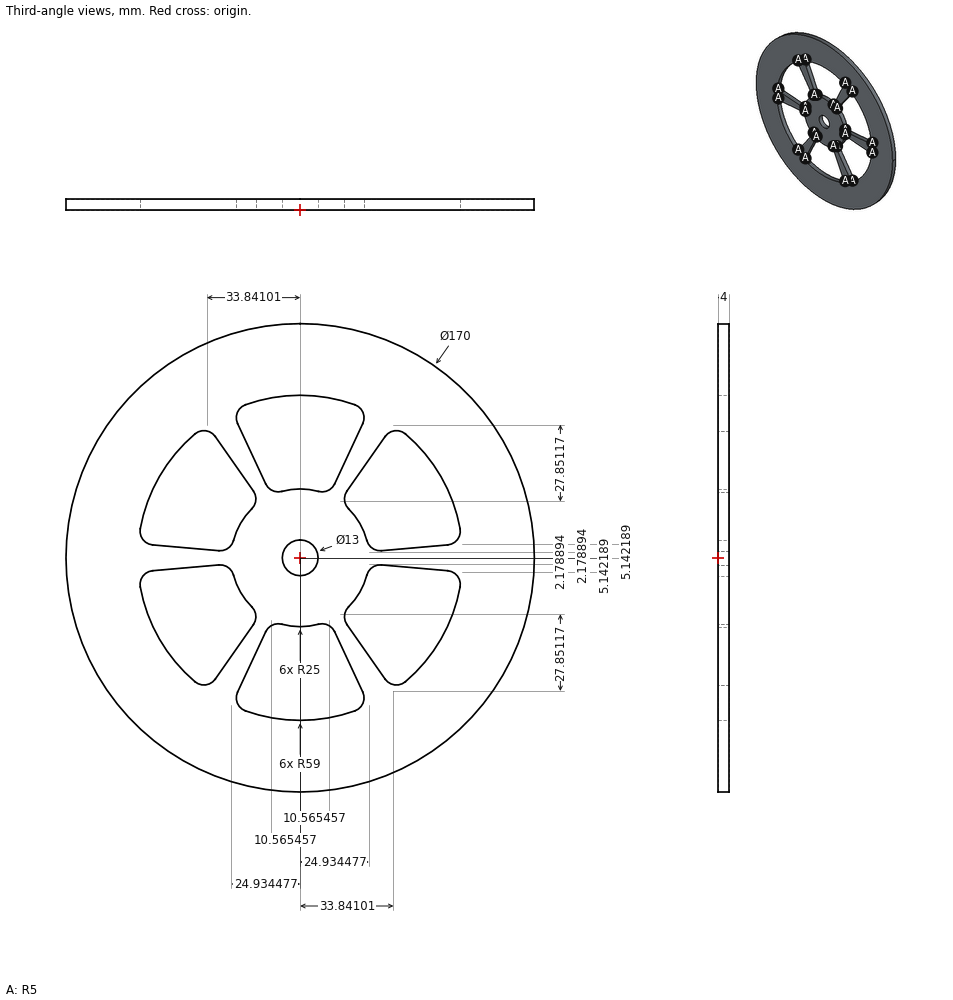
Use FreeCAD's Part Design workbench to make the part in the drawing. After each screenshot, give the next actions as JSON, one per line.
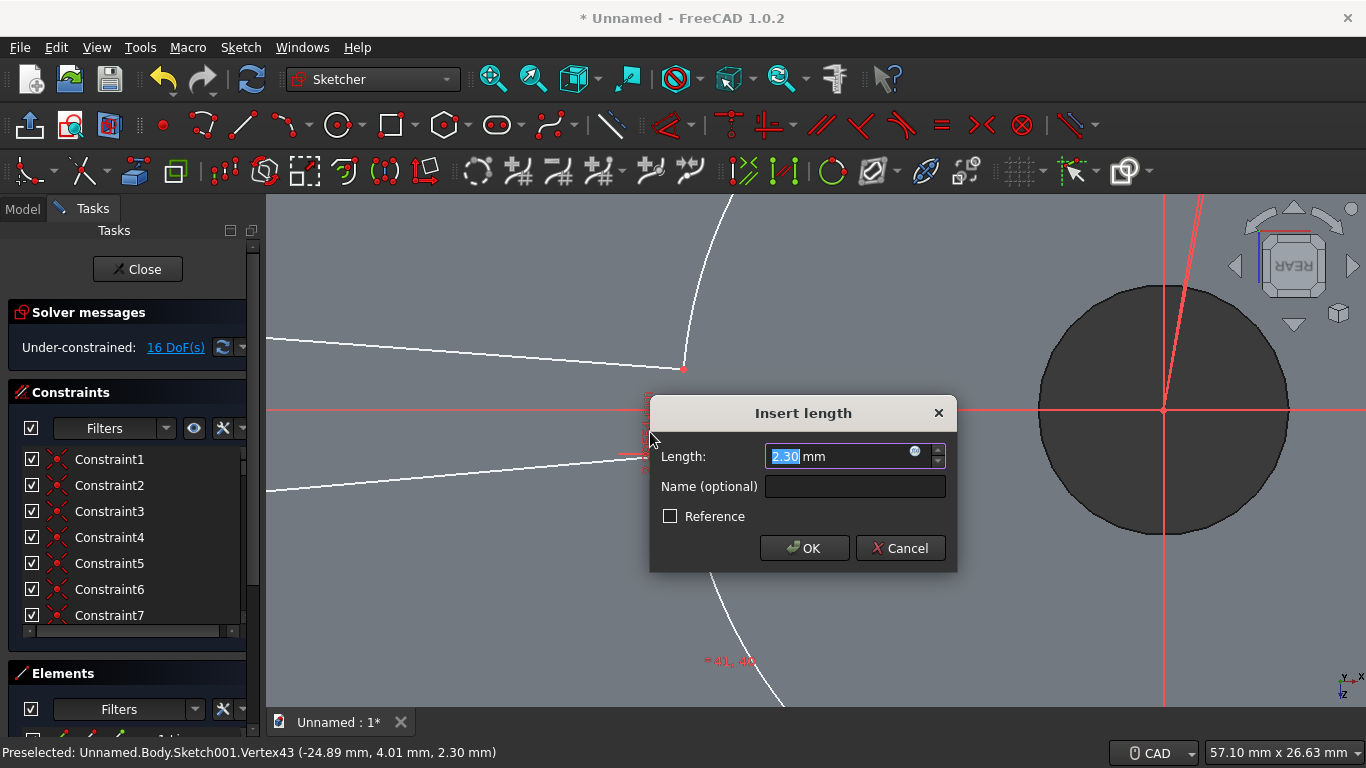
{"action": "type", "text": "2.178894"}
{"action": "key", "text": "Return"}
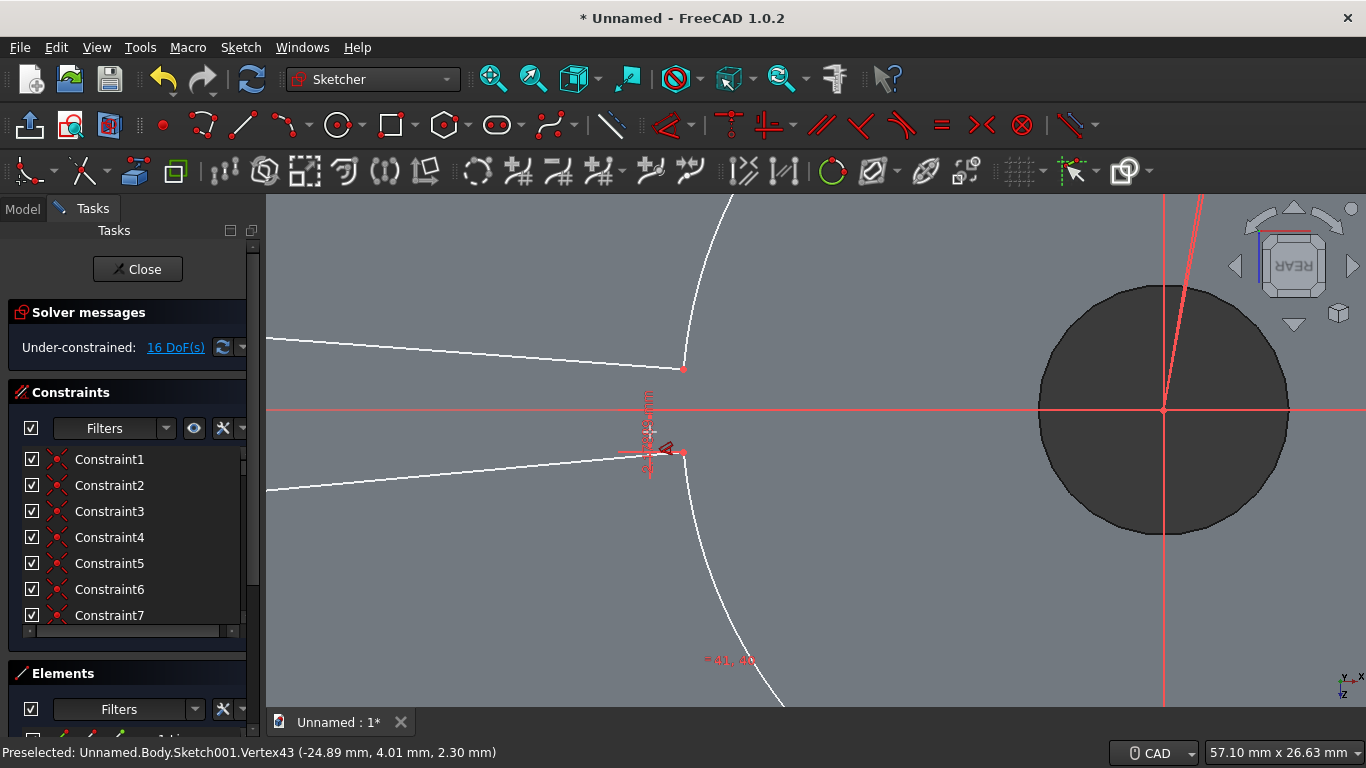
{"action": "scroll", "coordinate": [682, 457], "scroll_direction": "down", "scroll_amount": 10}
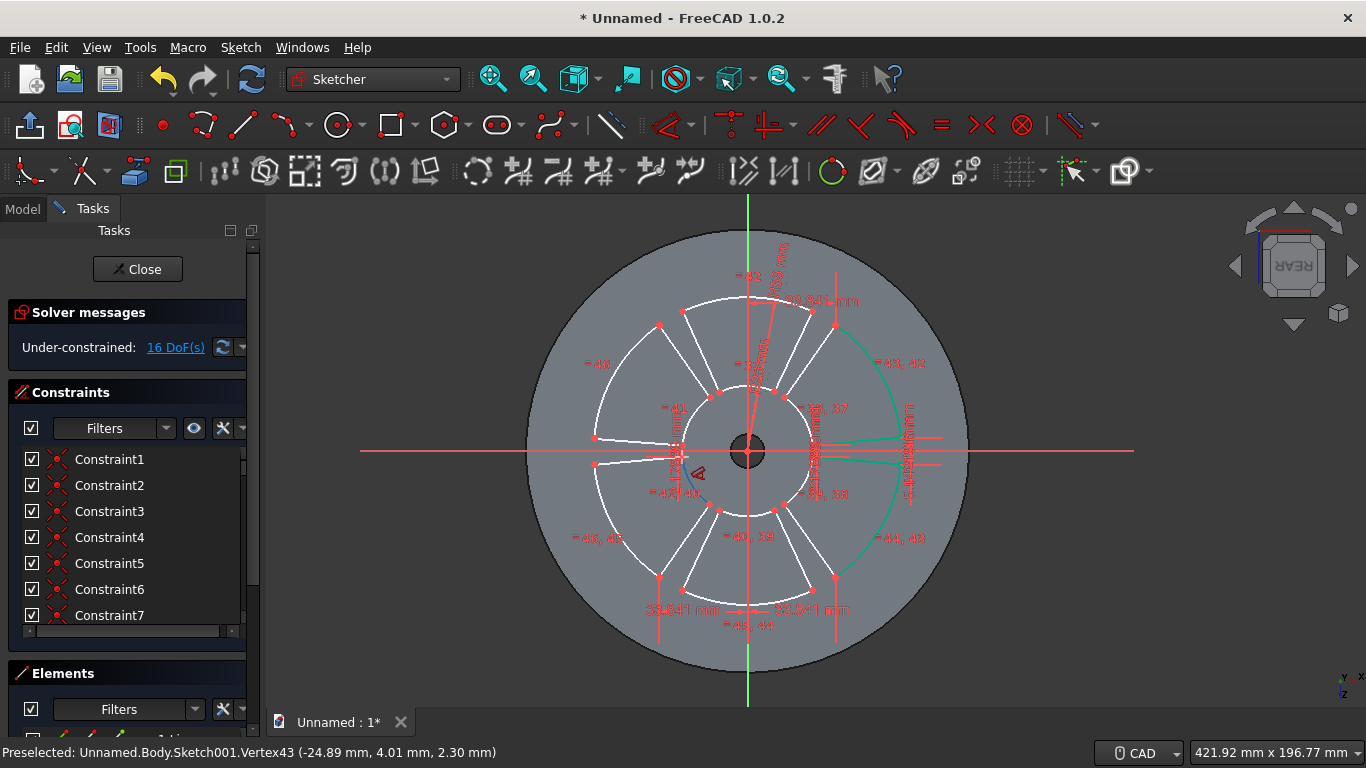
{"action": "scroll", "coordinate": [594, 465], "scroll_direction": "up", "scroll_amount": 6}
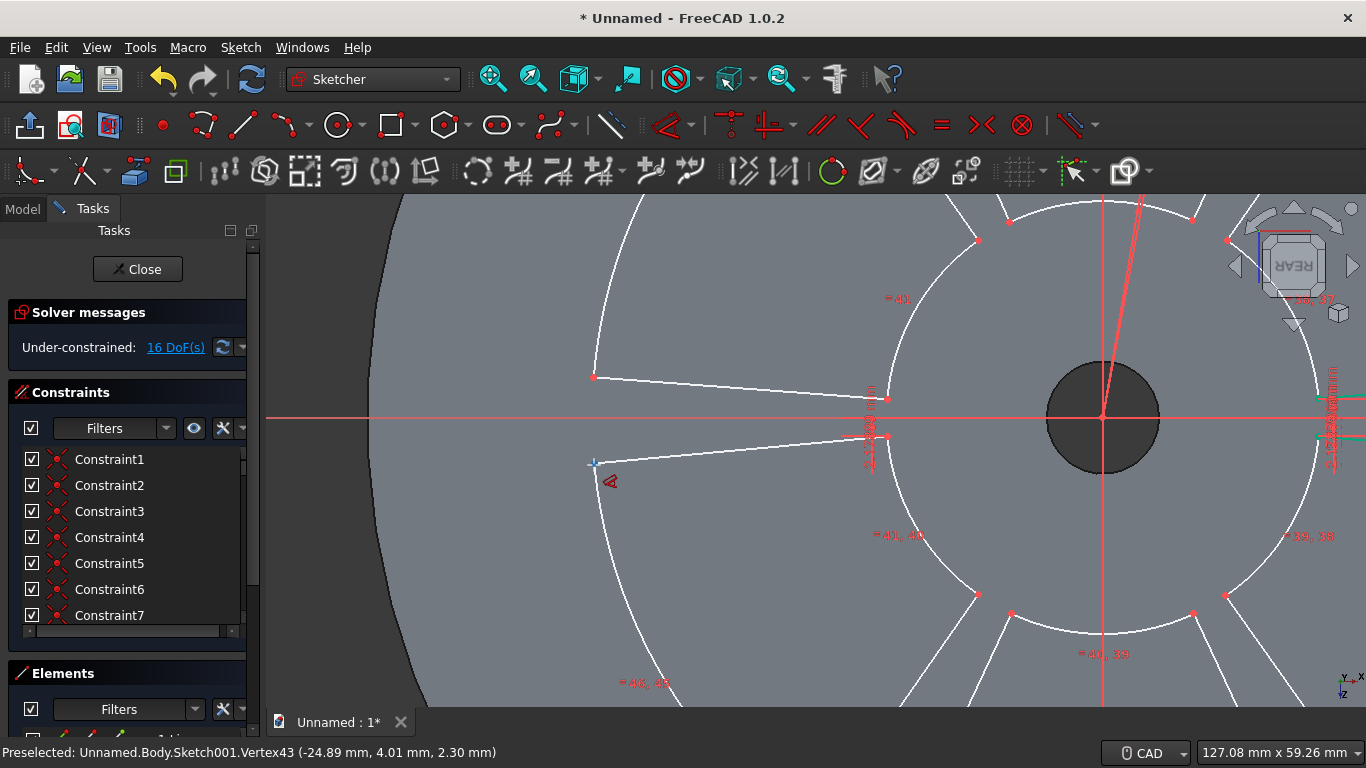
{"action": "left_click", "coordinate": [594, 463]}
{"action": "left_click", "coordinate": [560, 441]}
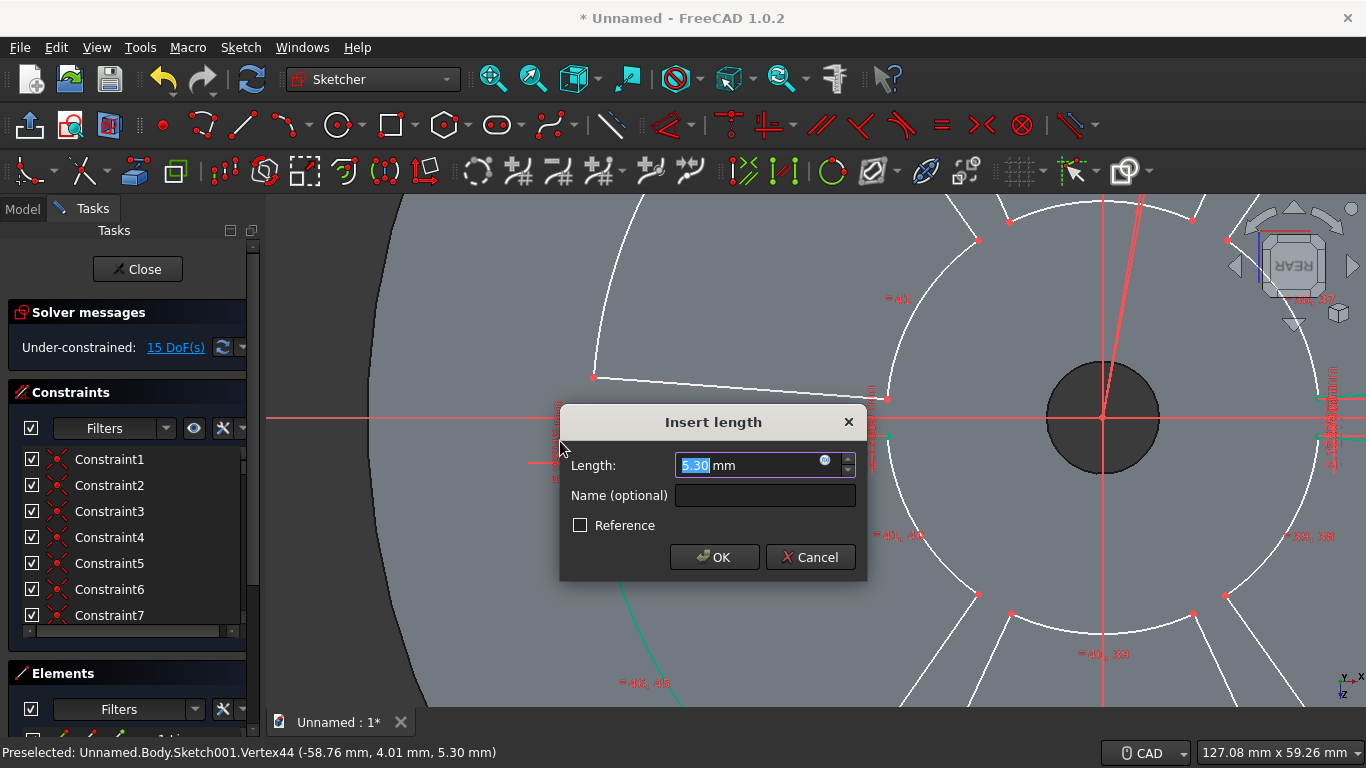
{"action": "type", "text": "5.142189"}
{"action": "key", "text": "Return"}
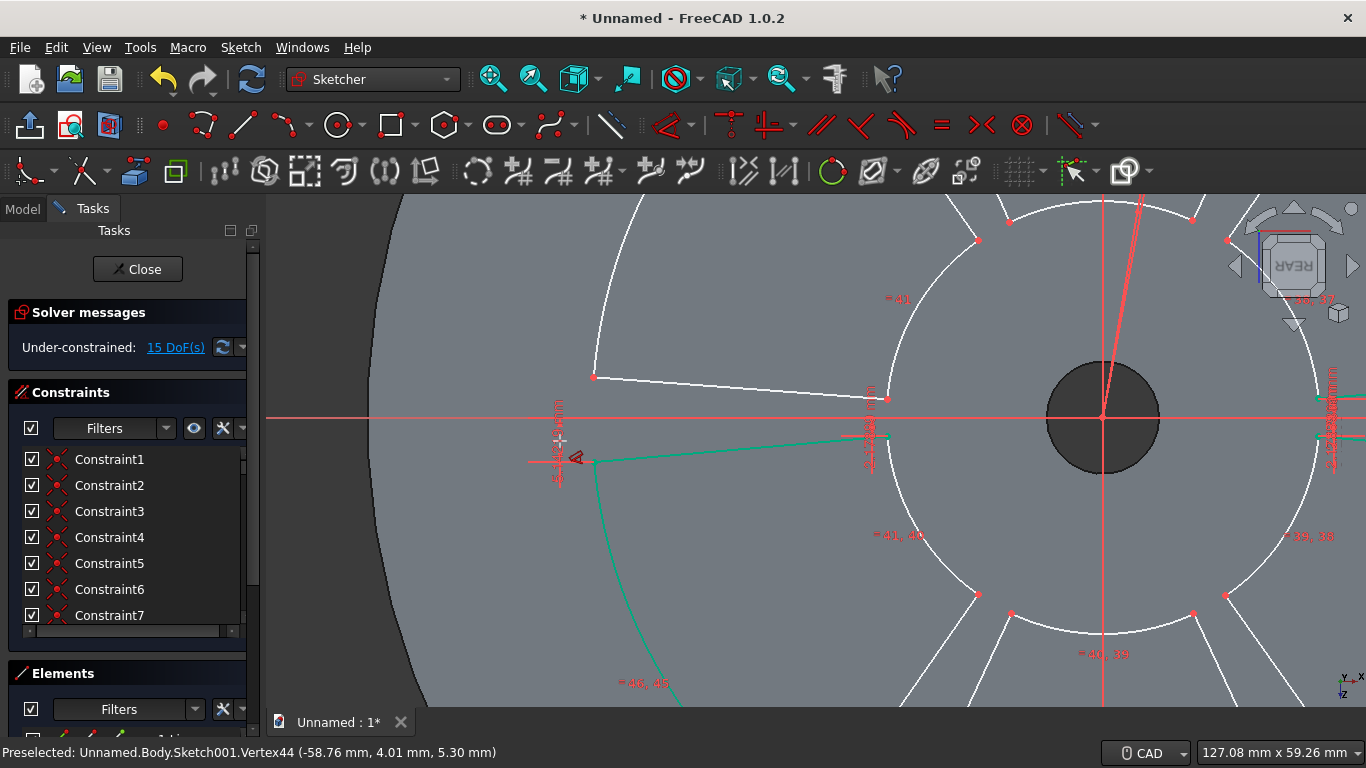
{"action": "left_click", "coordinate": [594, 377]}
{"action": "left_click", "coordinate": [560, 397]}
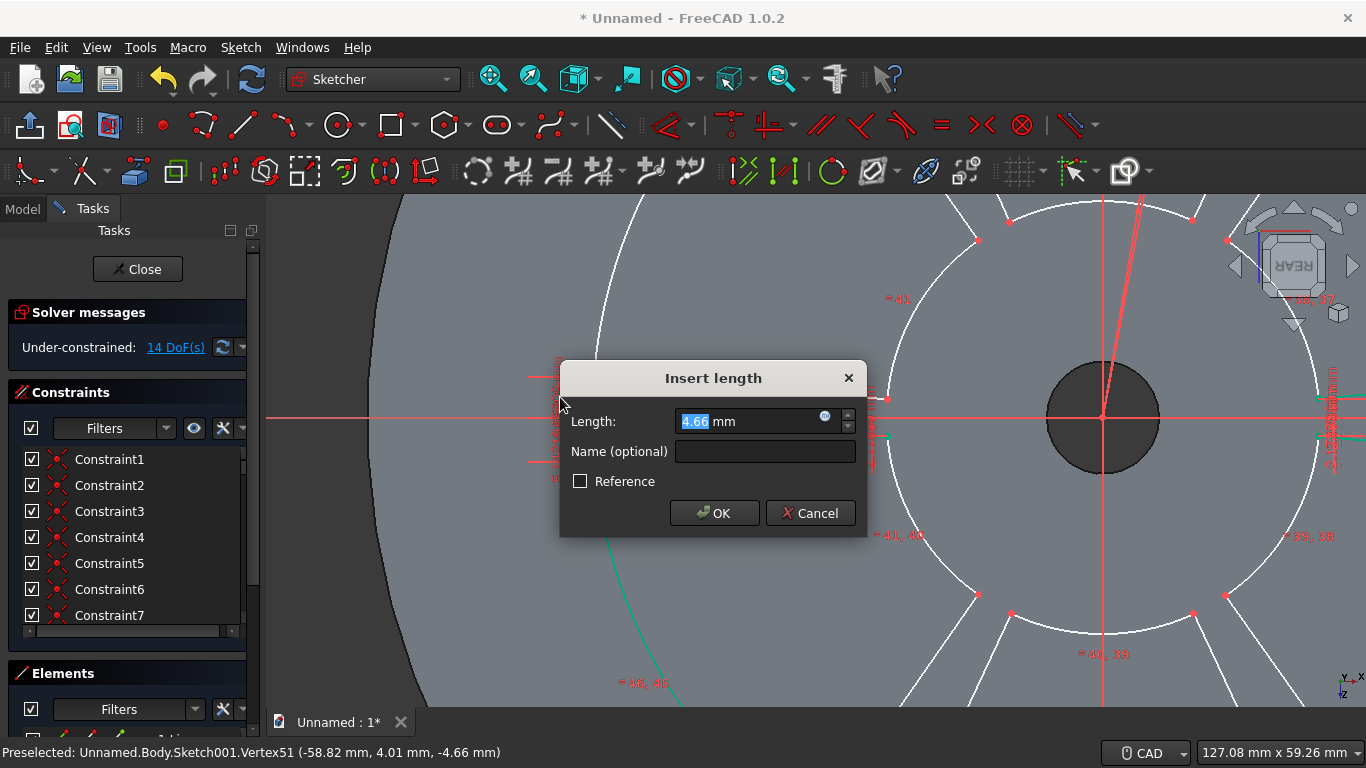
{"action": "type", "text": "5.142189"}
{"action": "key", "text": "Return"}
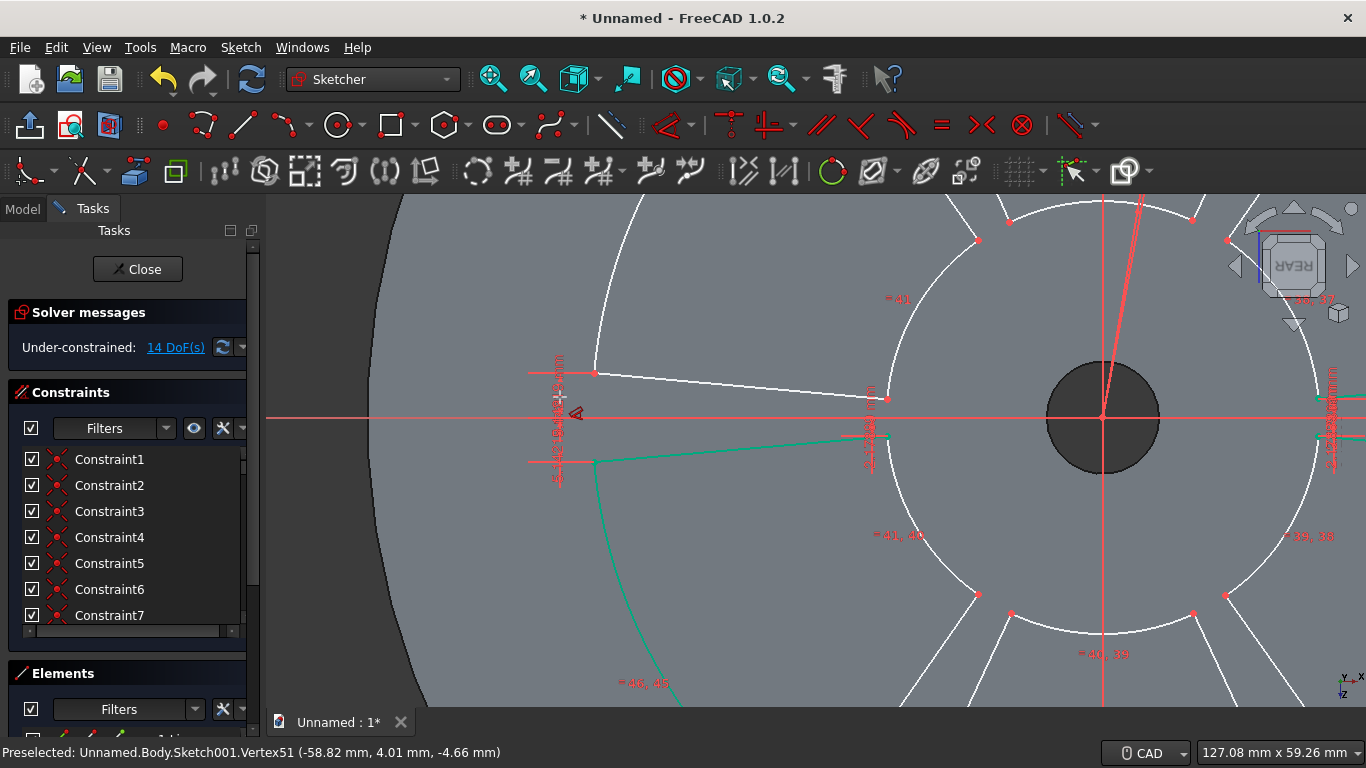
{"action": "scroll", "coordinate": [887, 399], "scroll_direction": "up", "scroll_amount": 4}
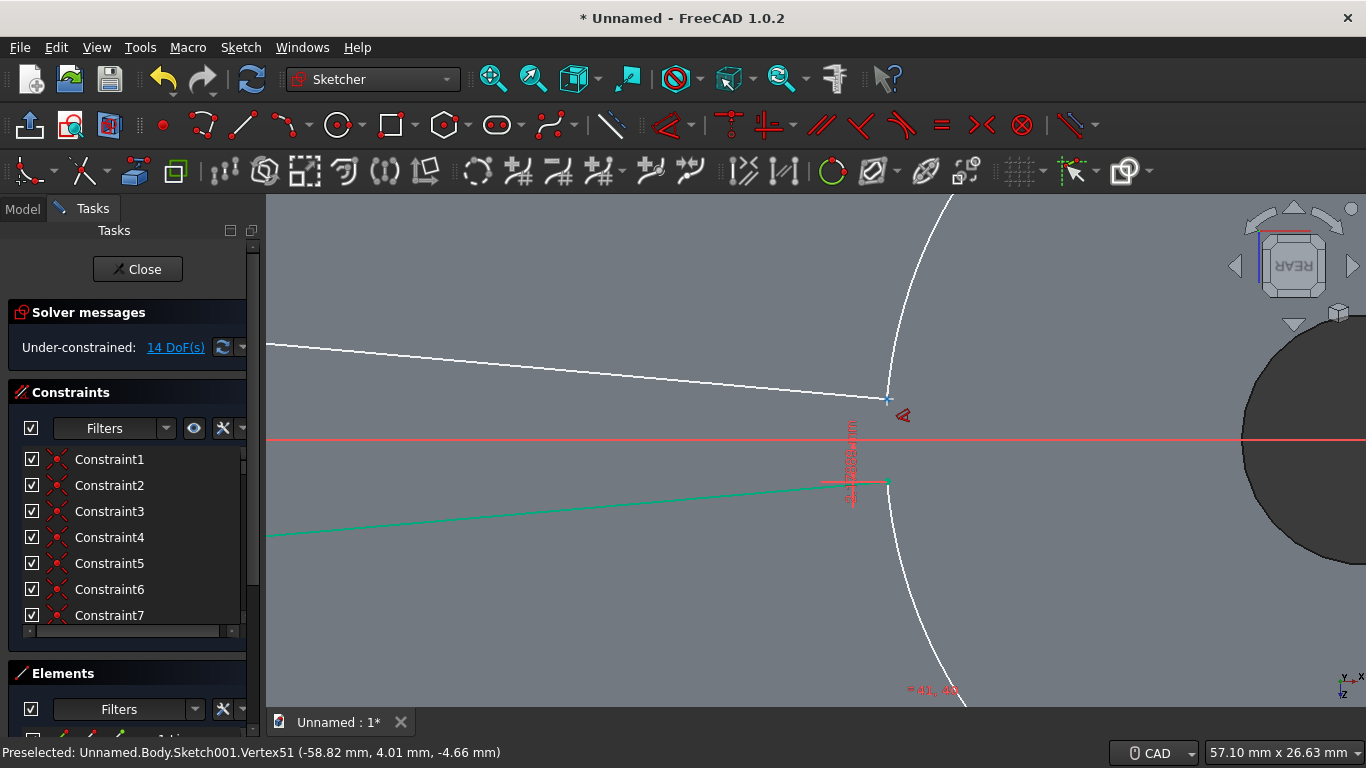
{"action": "left_click", "coordinate": [887, 399]}
{"action": "left_click", "coordinate": [853, 420]}